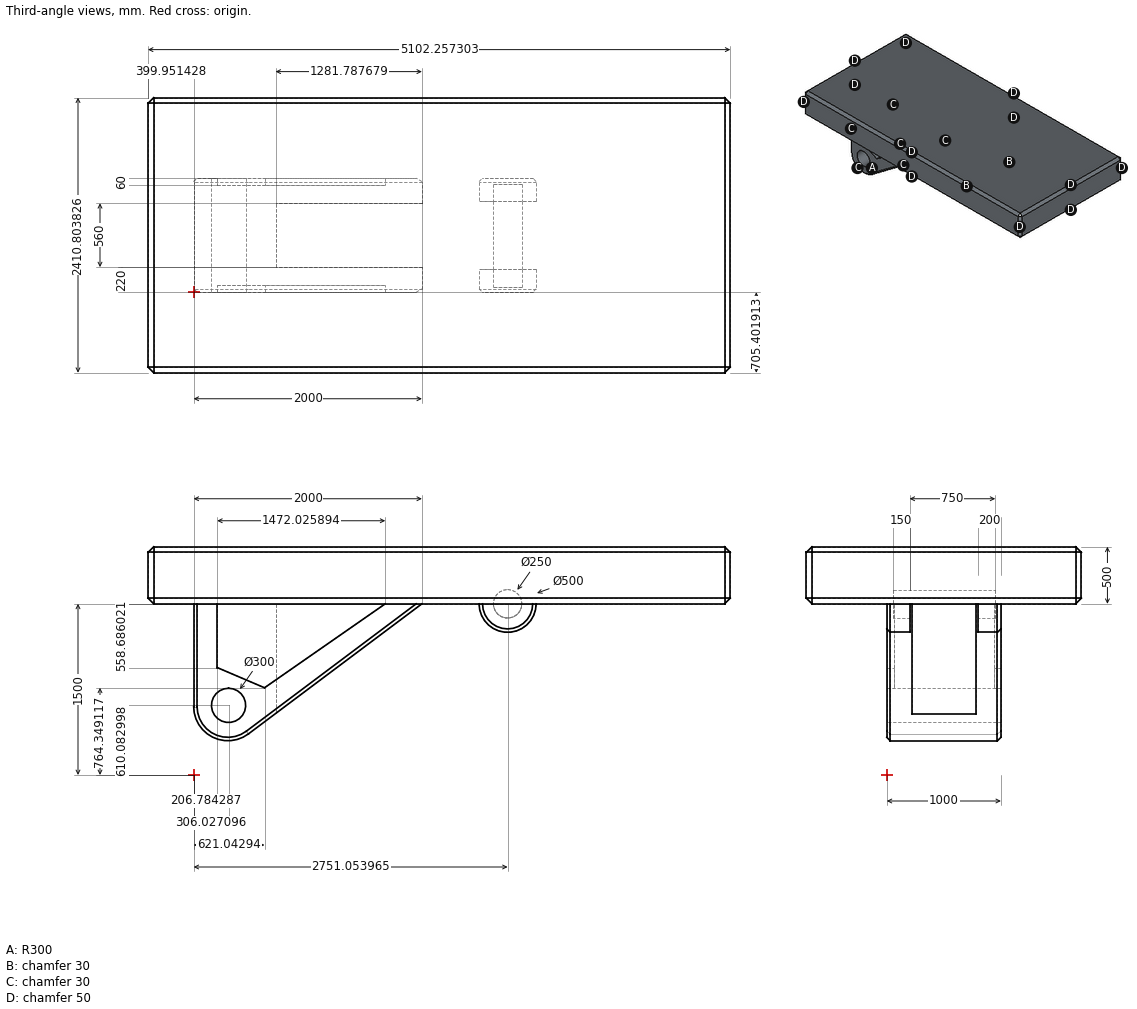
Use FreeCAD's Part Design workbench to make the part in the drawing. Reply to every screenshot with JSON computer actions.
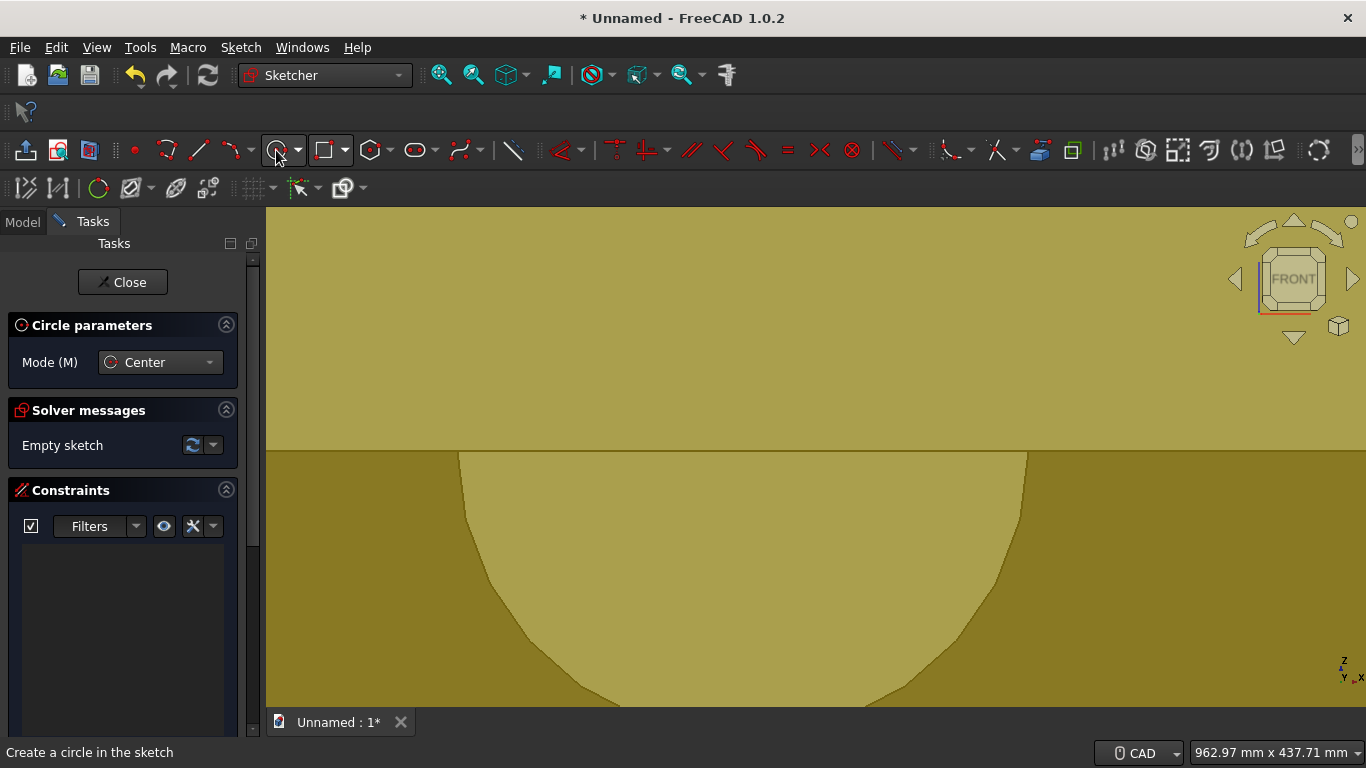
{"action": "left_click", "coordinate": [743, 451]}
{"action": "mouse_move", "coordinate": [844, 350]}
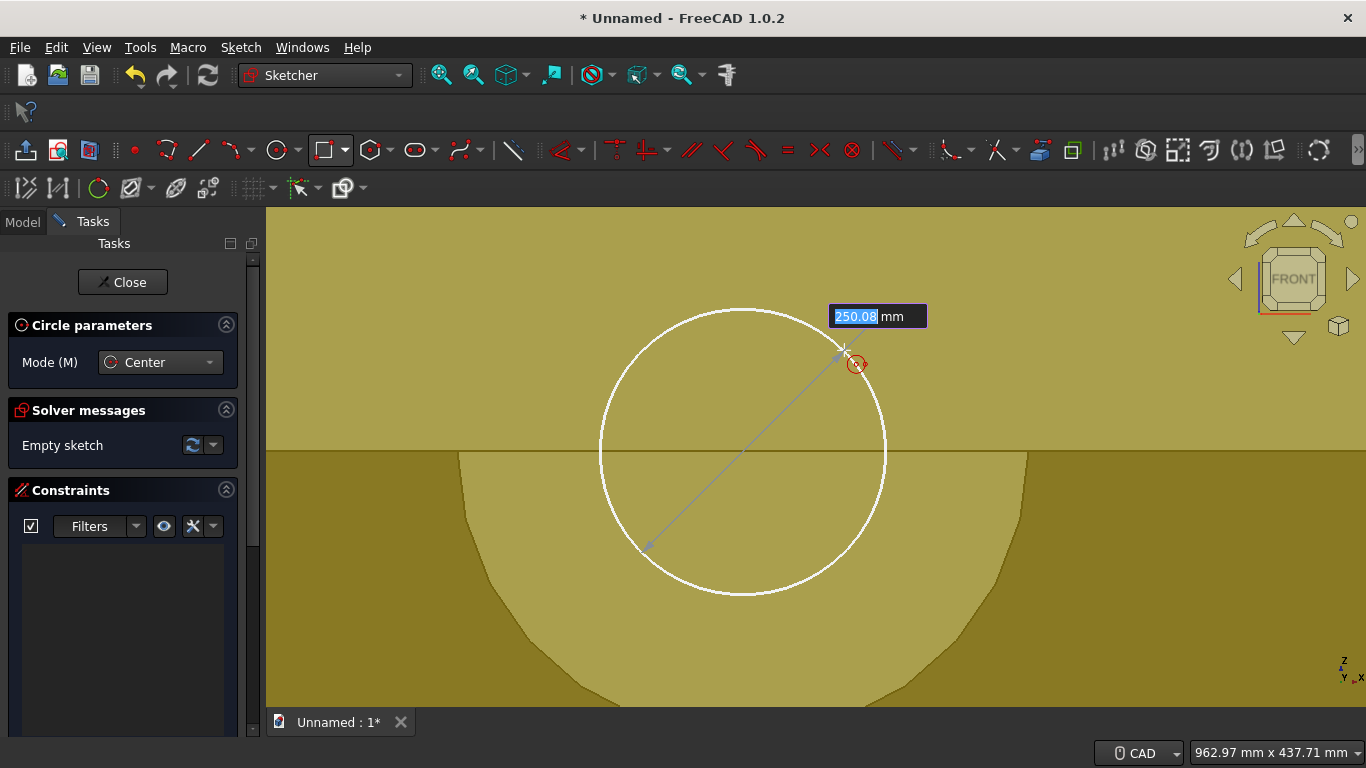
{"action": "type", "text": "250"}
{"action": "key", "text": "Return"}
{"action": "key", "text": "Escape"}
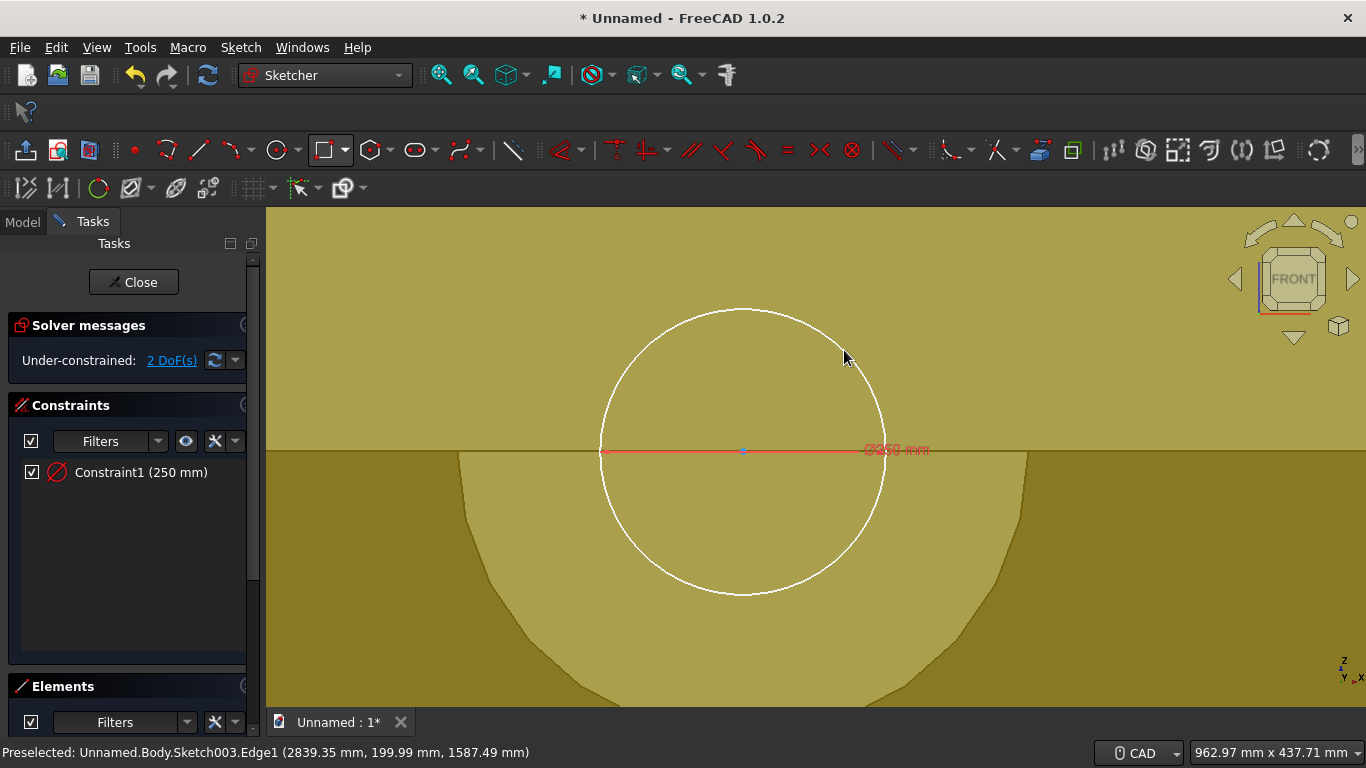
{"action": "left_click", "coordinate": [560, 150]}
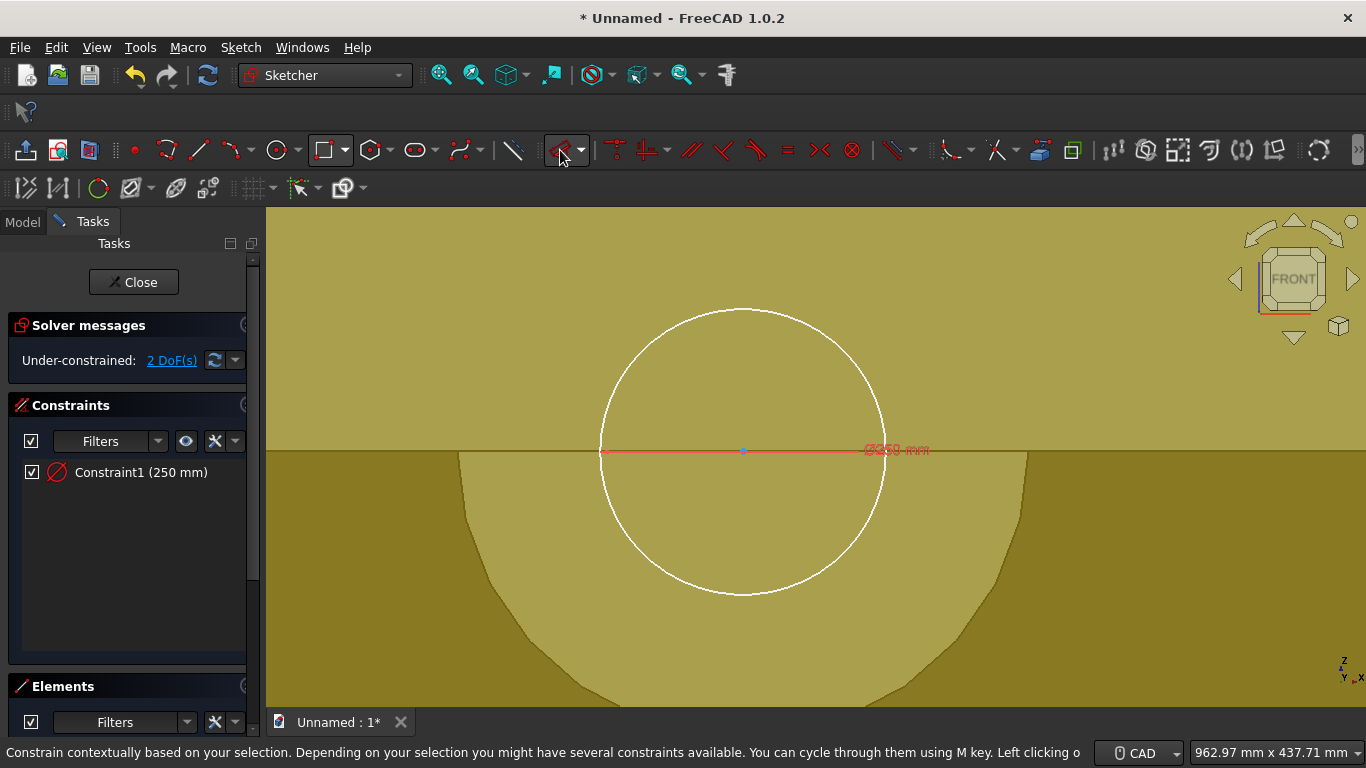
{"action": "left_click", "coordinate": [743, 452]}
{"action": "left_click", "coordinate": [777, 566]}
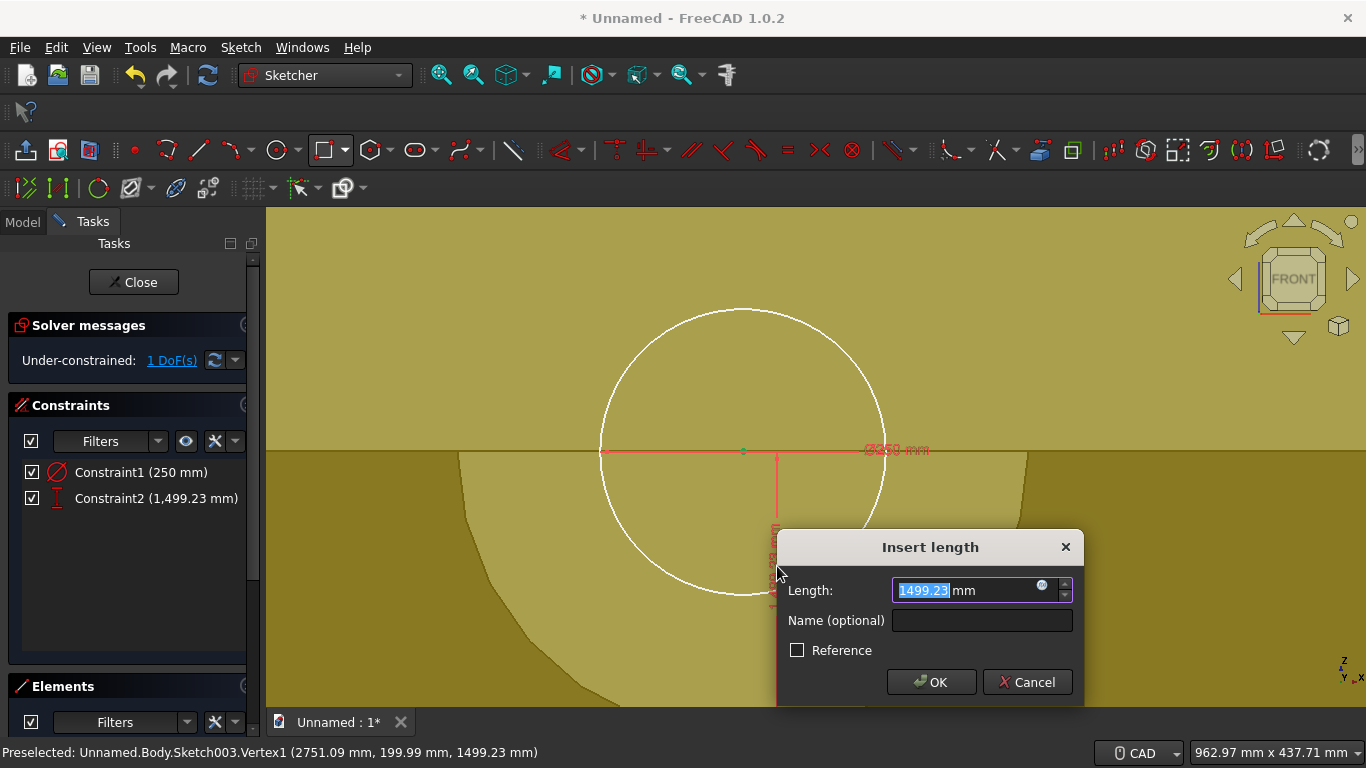
{"action": "type", "text": "1500"}
{"action": "key", "text": "Return"}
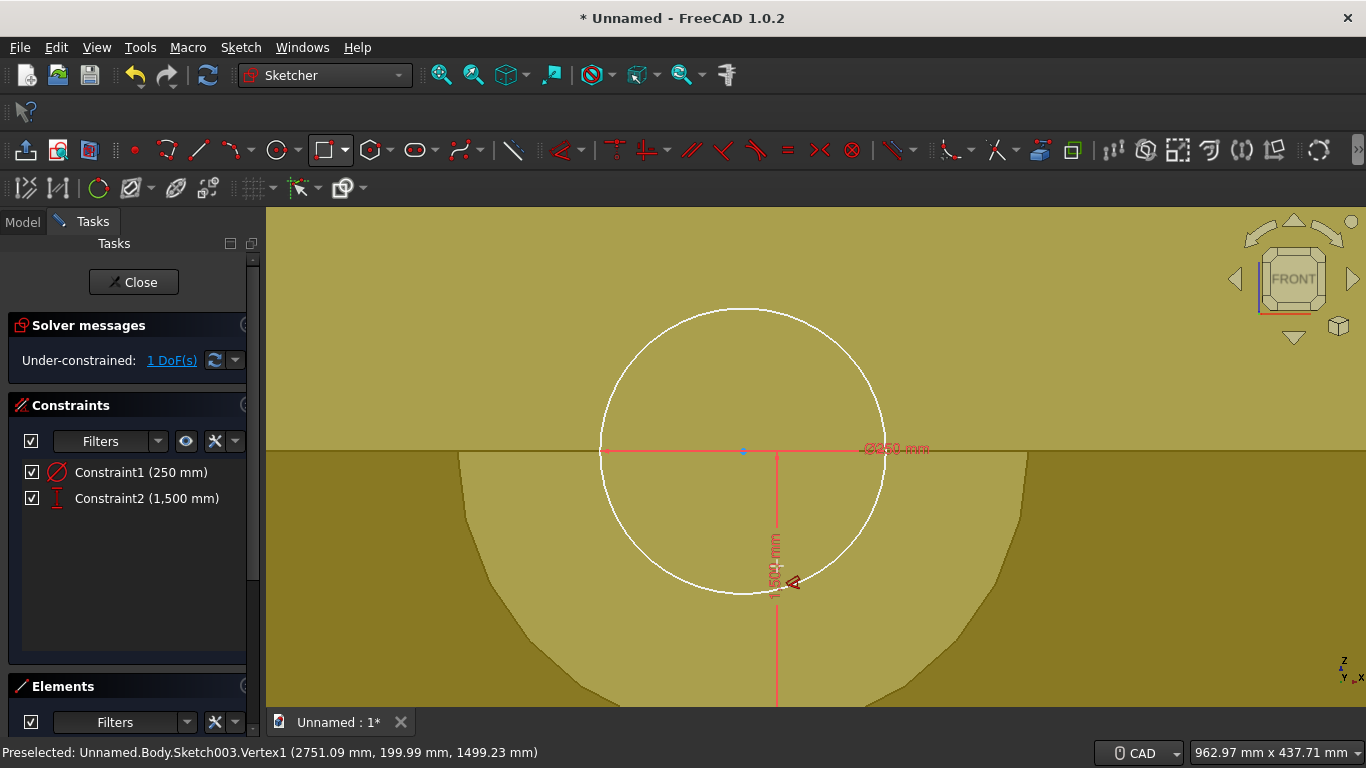
{"action": "left_click", "coordinate": [743, 451]}
{"action": "left_click", "coordinate": [519, 417]}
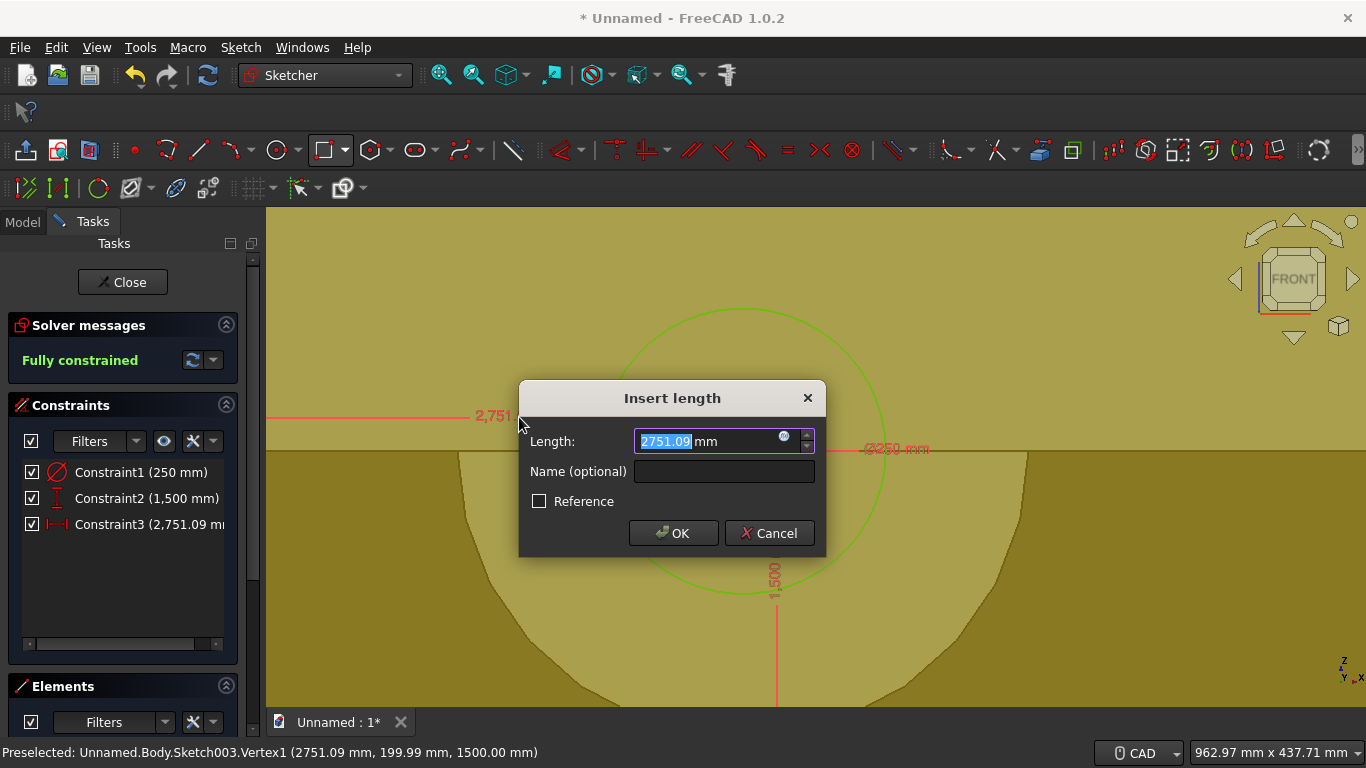
{"action": "type", "text": "2751.053965"}
{"action": "key", "text": "Return"}
{"action": "key", "text": "Escape"}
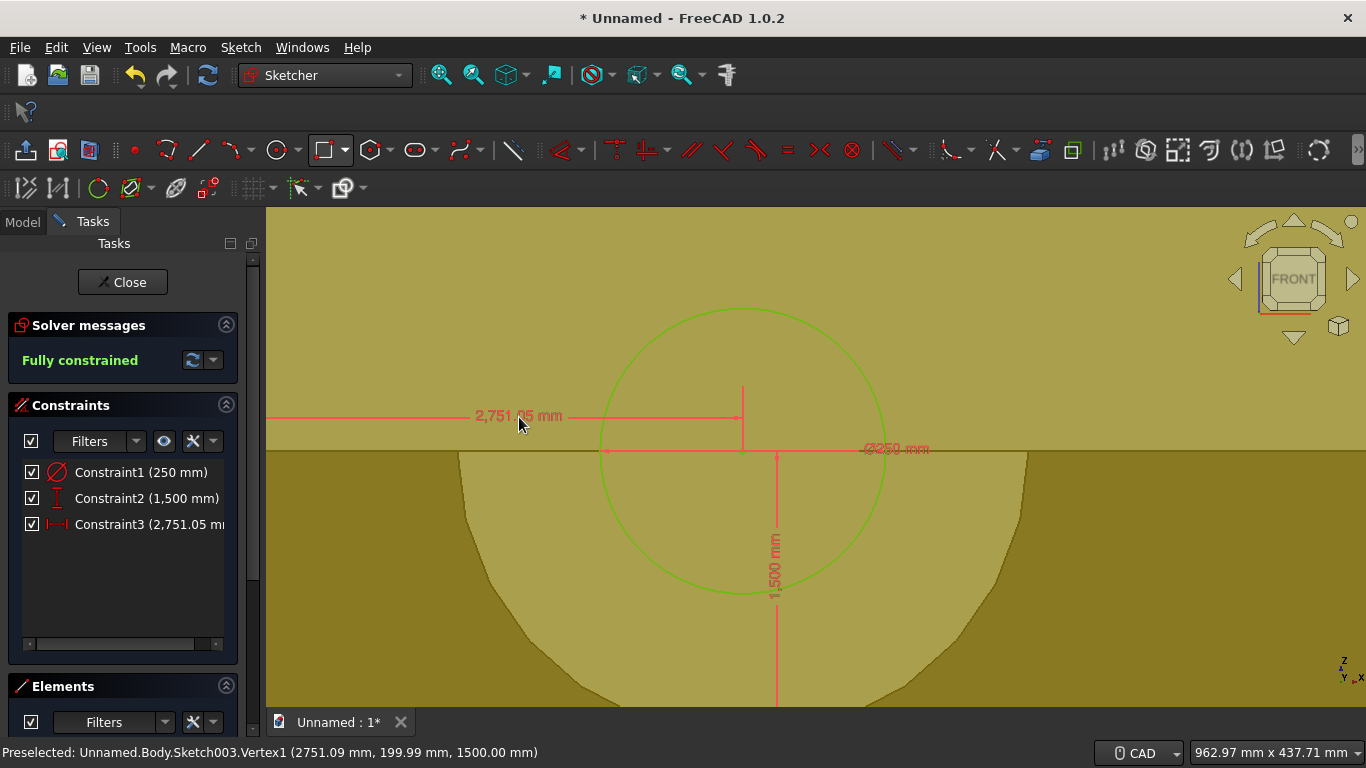
{"action": "left_click", "coordinate": [123, 282]}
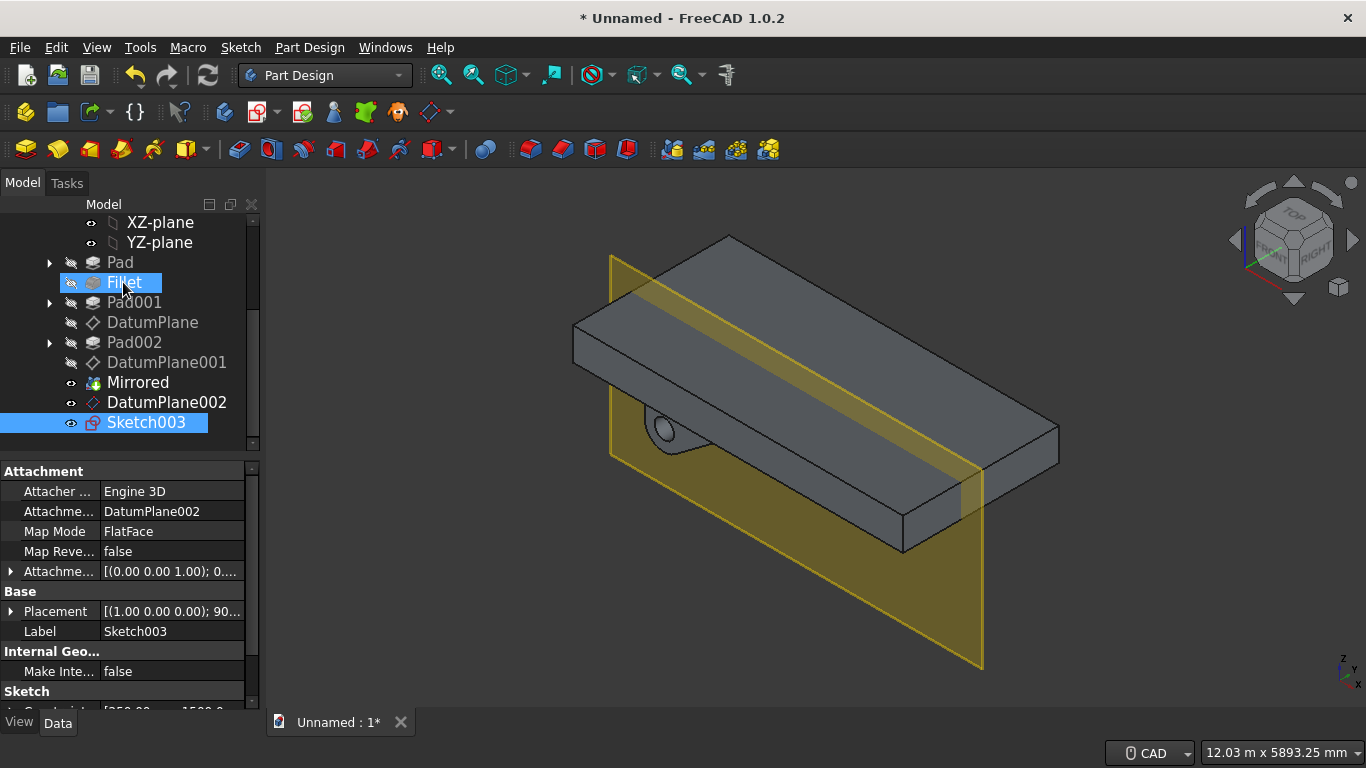
{"action": "left_click", "coordinate": [240, 150]}